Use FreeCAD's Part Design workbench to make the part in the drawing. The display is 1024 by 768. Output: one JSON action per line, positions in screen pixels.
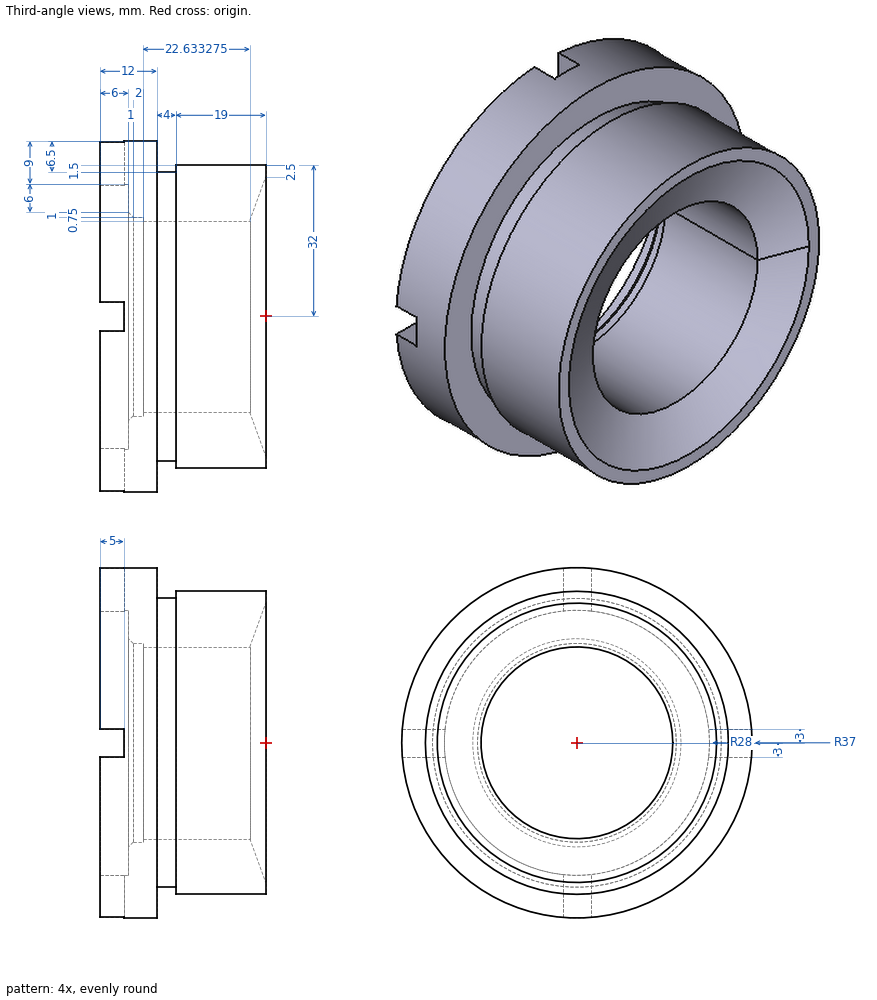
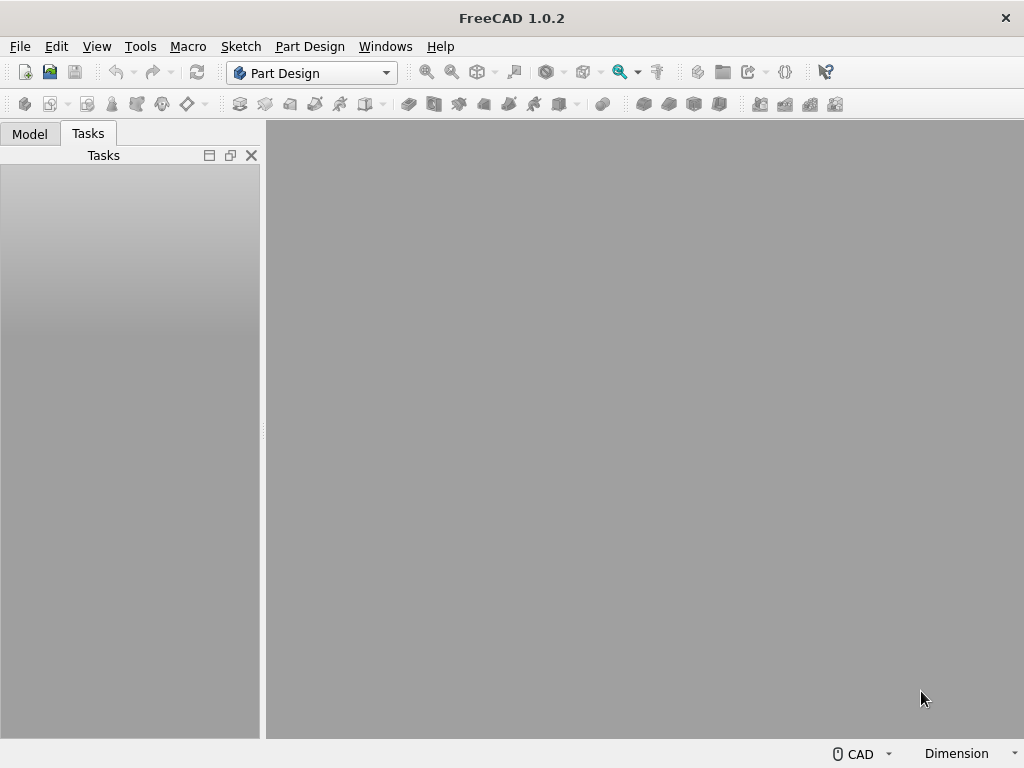
{"action": "left_click", "coordinate": [25, 72]}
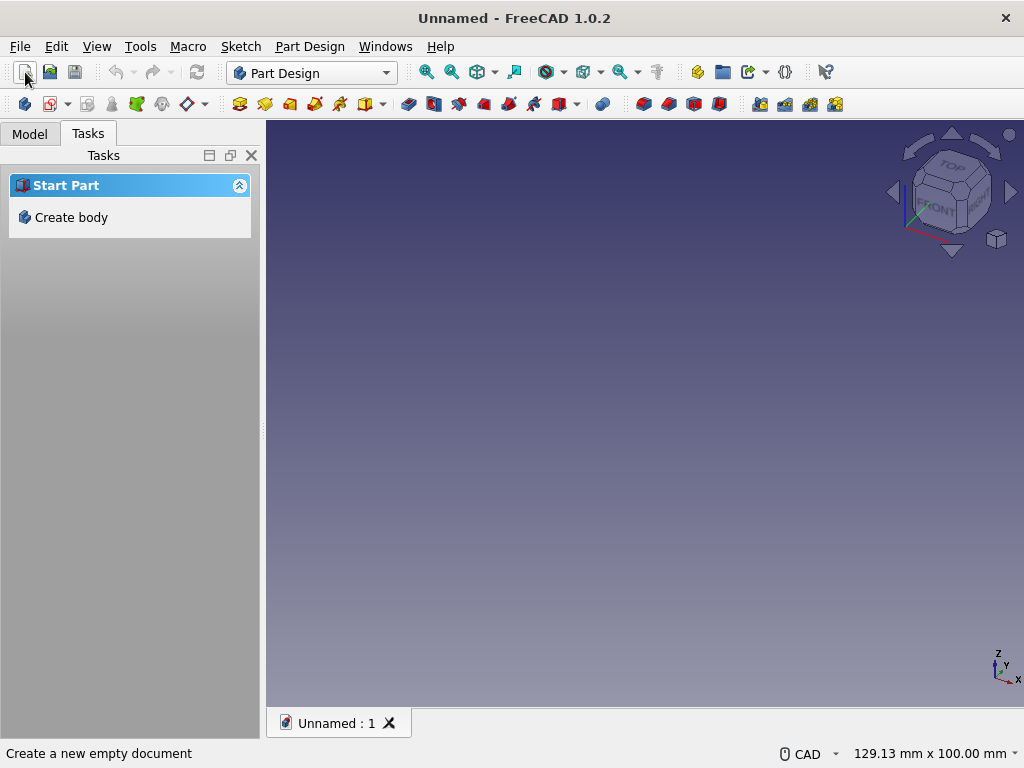
{"action": "left_click", "coordinate": [50, 104]}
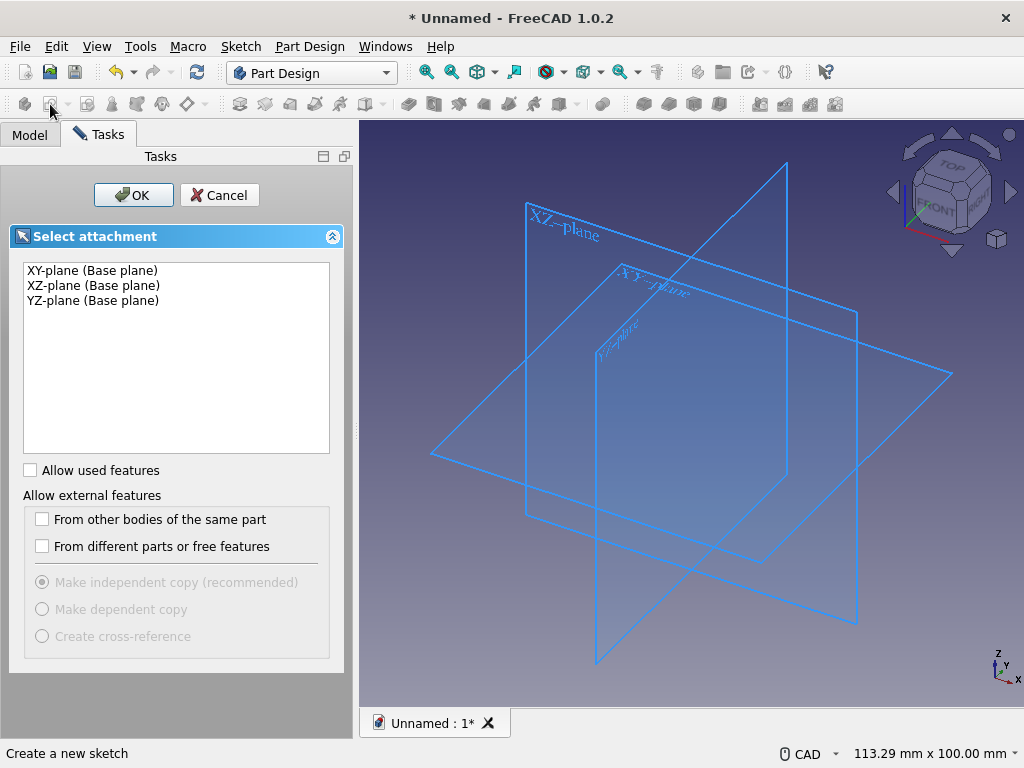
{"action": "left_click", "coordinate": [84, 270]}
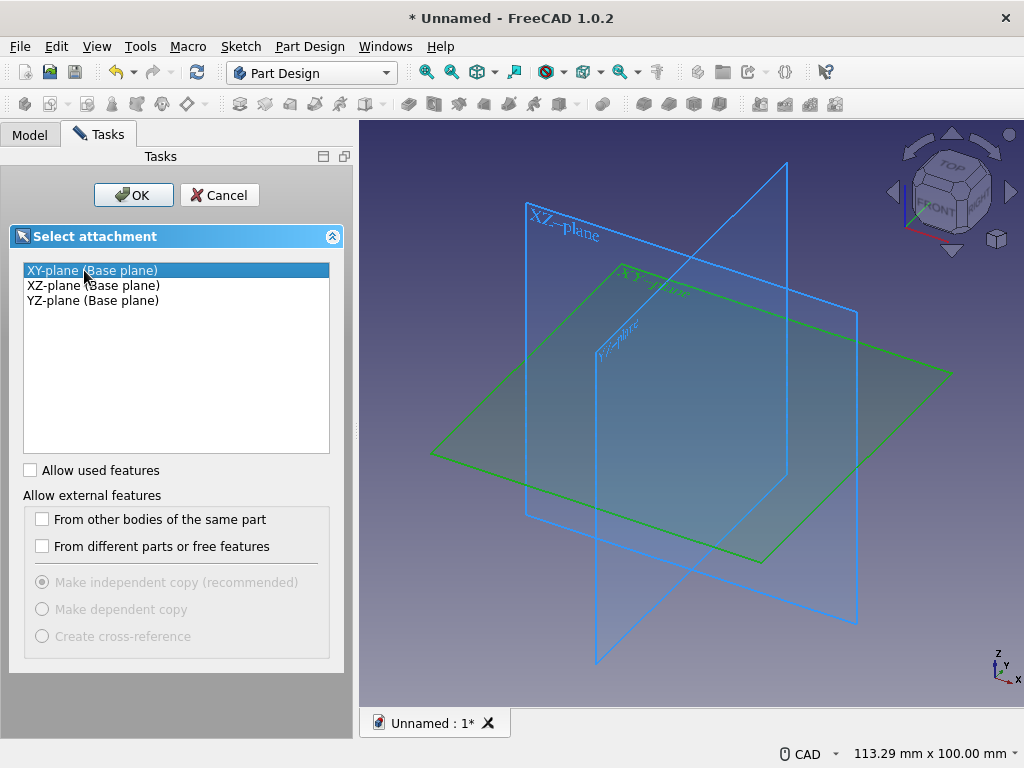
{"action": "left_click", "coordinate": [134, 195]}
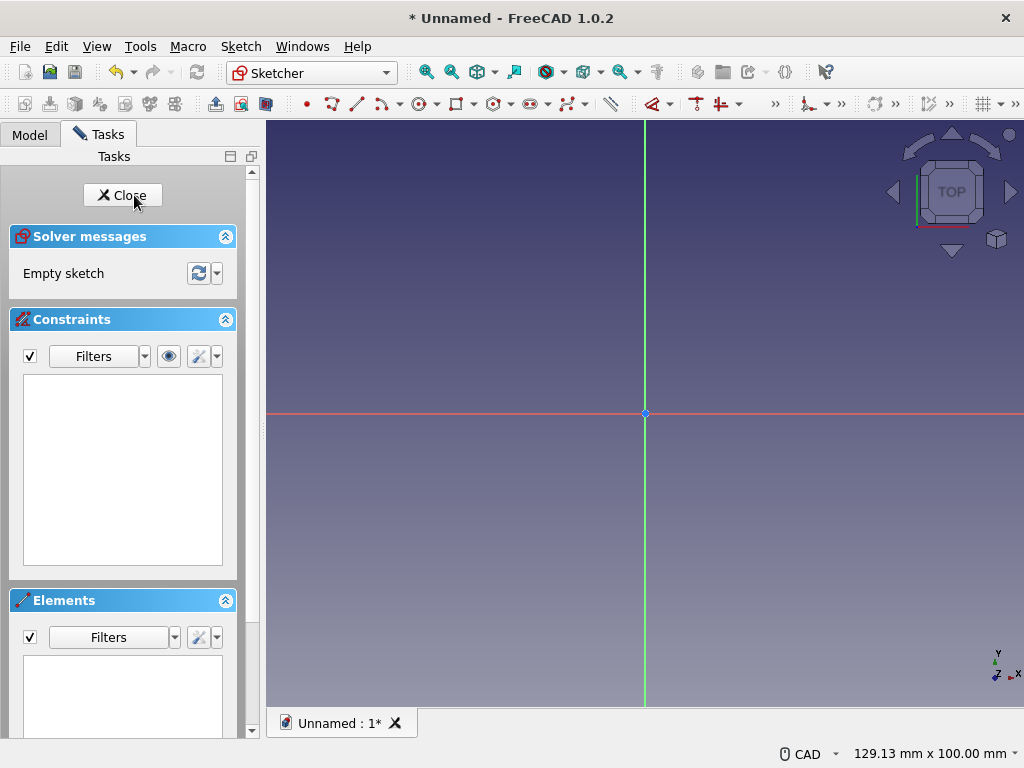
{"action": "scroll", "coordinate": [501, 173], "scroll_direction": "up", "scroll_amount": 3}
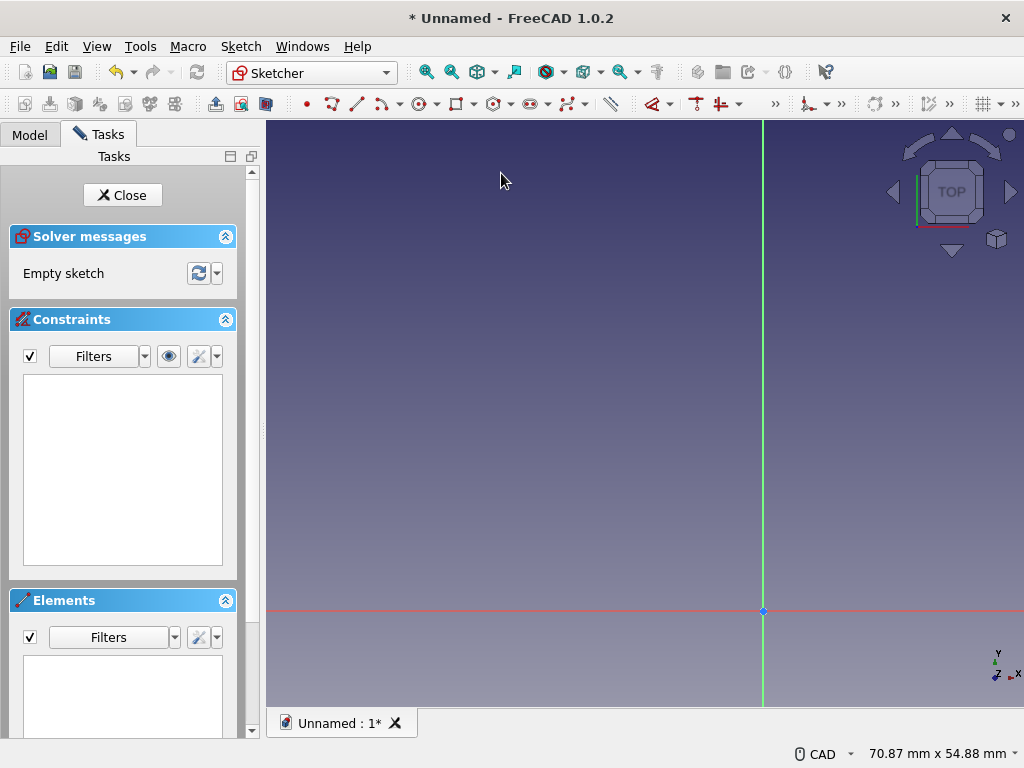
{"action": "left_click", "coordinate": [332, 104]}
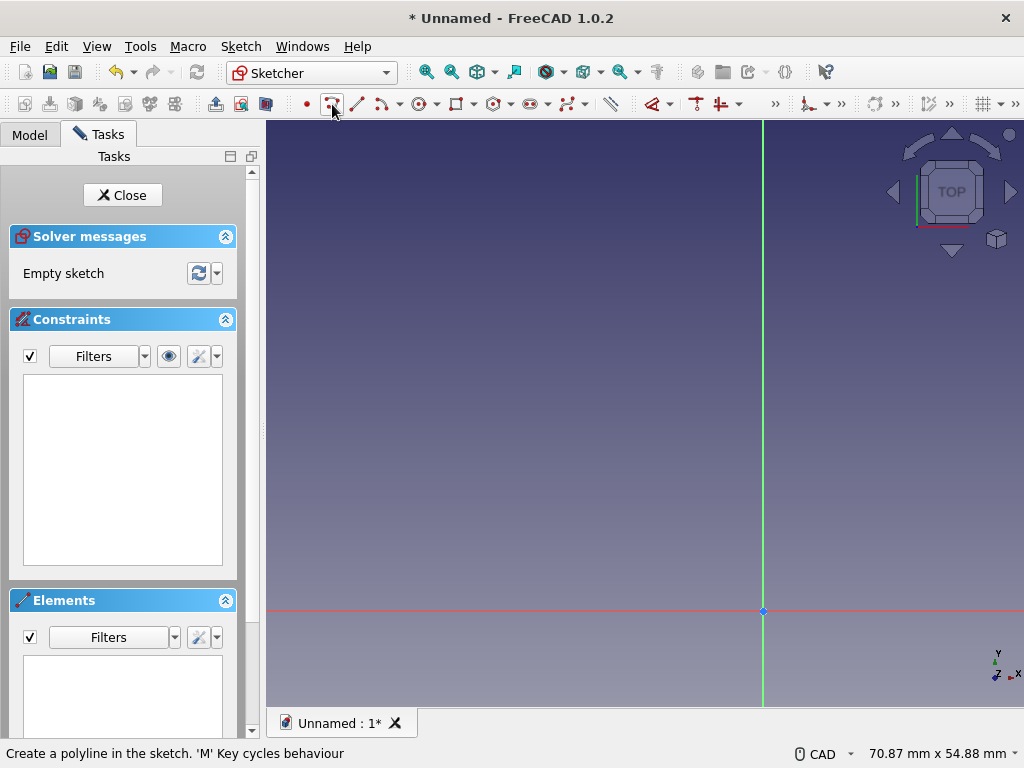
{"action": "left_click", "coordinate": [727, 395]}
{"action": "left_click", "coordinate": [763, 296]}
{"action": "left_click", "coordinate": [754, 269]}
{"action": "left_click", "coordinate": [560, 269]}
{"action": "left_click", "coordinate": [560, 285]}
{"action": "left_click", "coordinate": [517, 285]}
{"action": "left_click", "coordinate": [517, 215]}
{"action": "left_click", "coordinate": [389, 215]}
{"action": "left_click", "coordinate": [389, 312]}
{"action": "left_click", "coordinate": [453, 312]}
{"action": "left_click", "coordinate": [453, 376]}
{"action": "left_click", "coordinate": [464, 387]}
{"action": "left_click", "coordinate": [485, 387]}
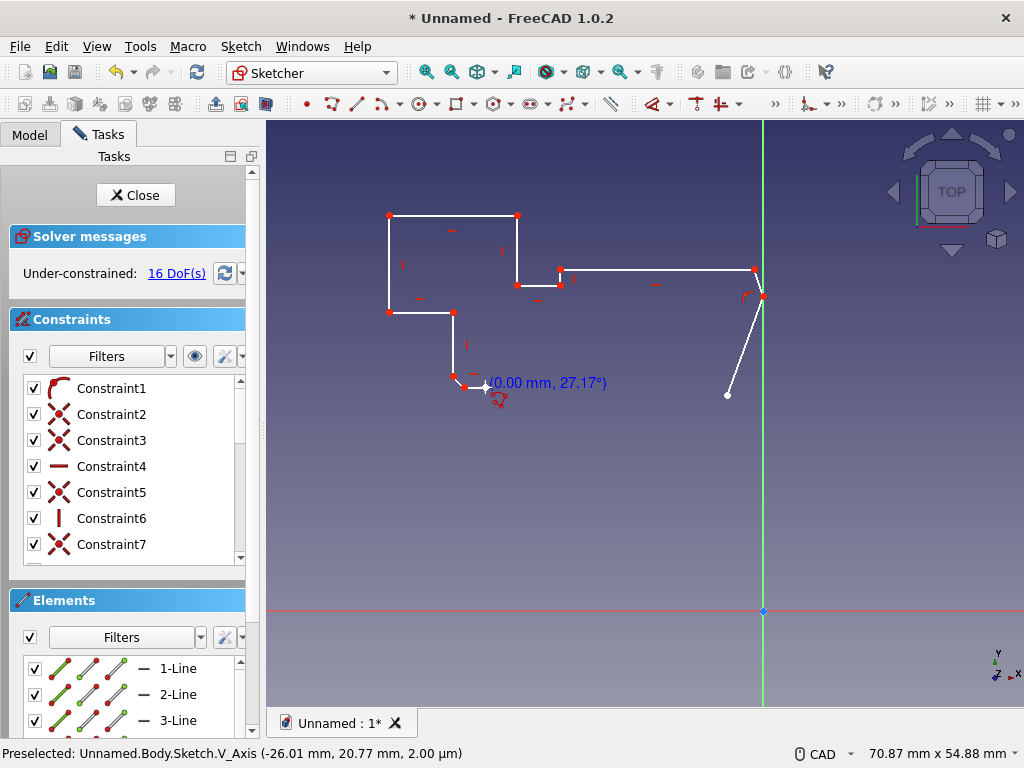
{"action": "scroll", "coordinate": [485, 395], "scroll_direction": "up", "scroll_amount": 4}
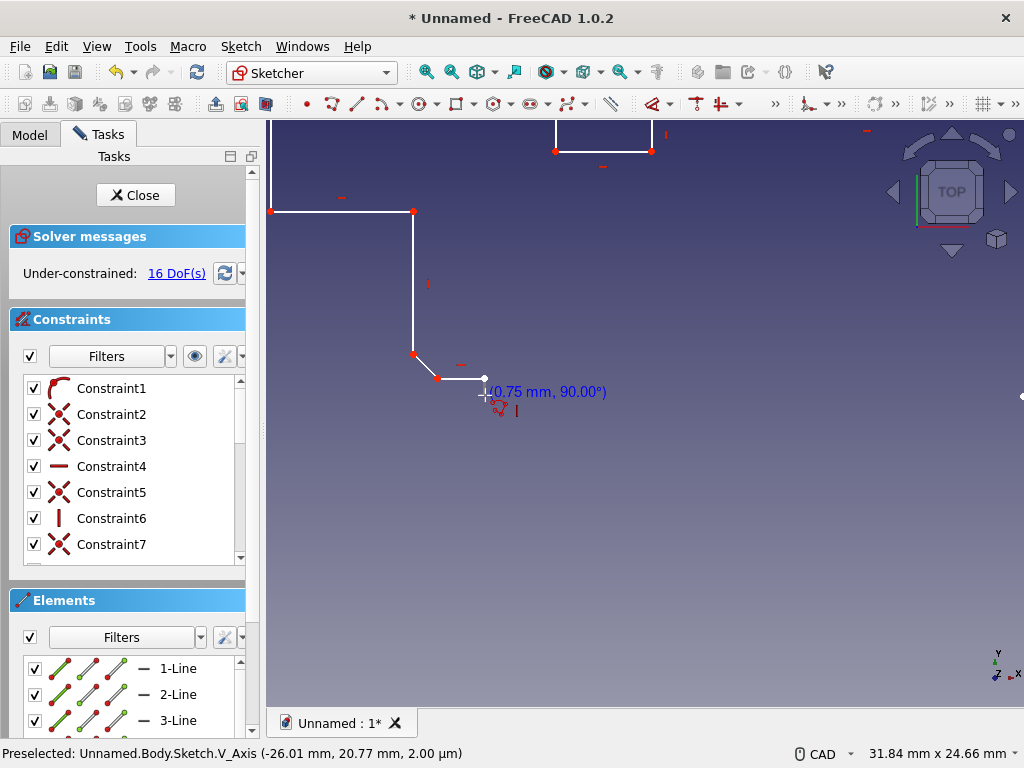
{"action": "left_click", "coordinate": [485, 393]}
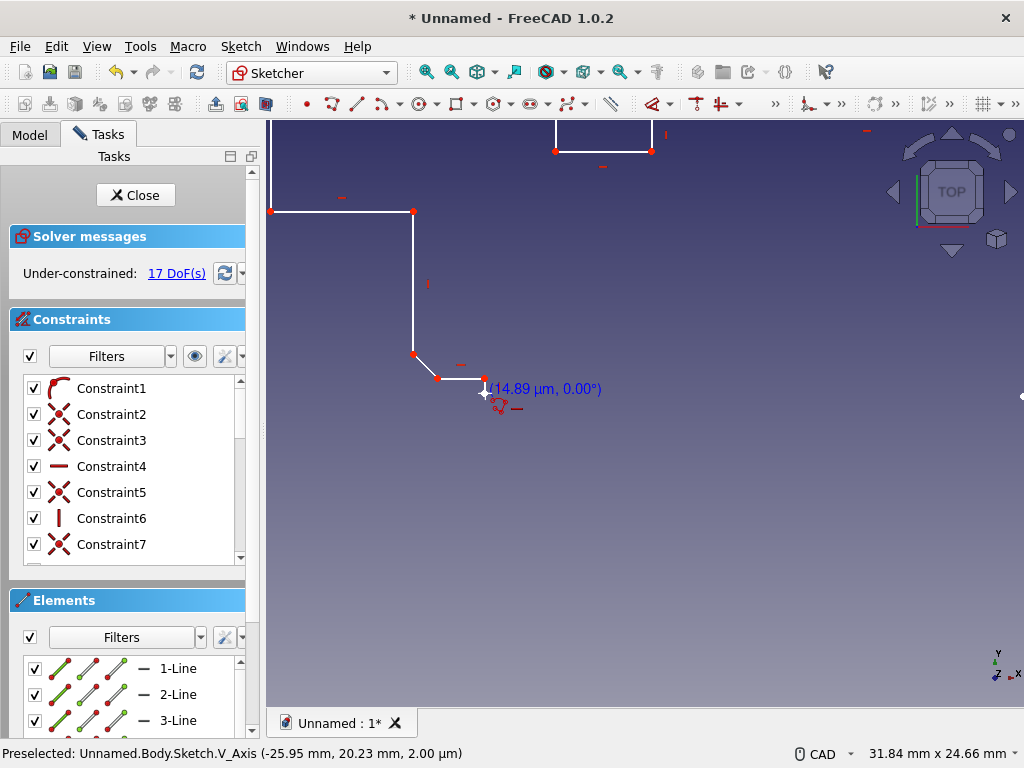
{"action": "scroll", "coordinate": [486, 396], "scroll_direction": "down", "scroll_amount": 4}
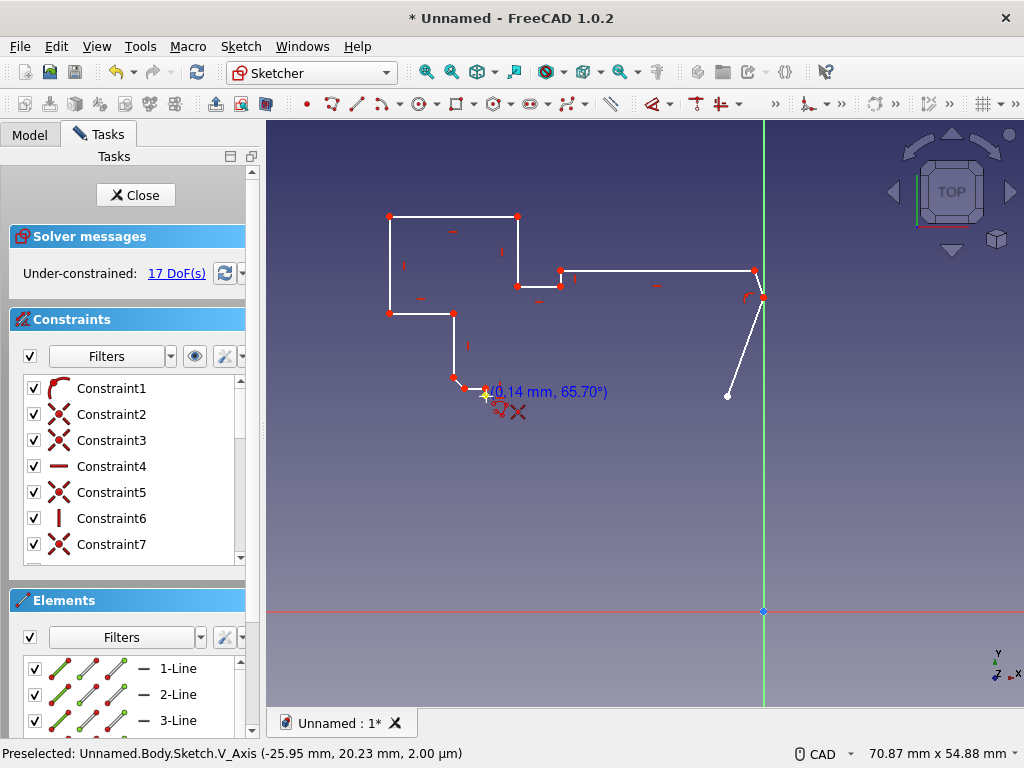
{"action": "left_click", "coordinate": [728, 397]}
{"action": "key", "text": "Escape"}
{"action": "key", "text": "Escape"}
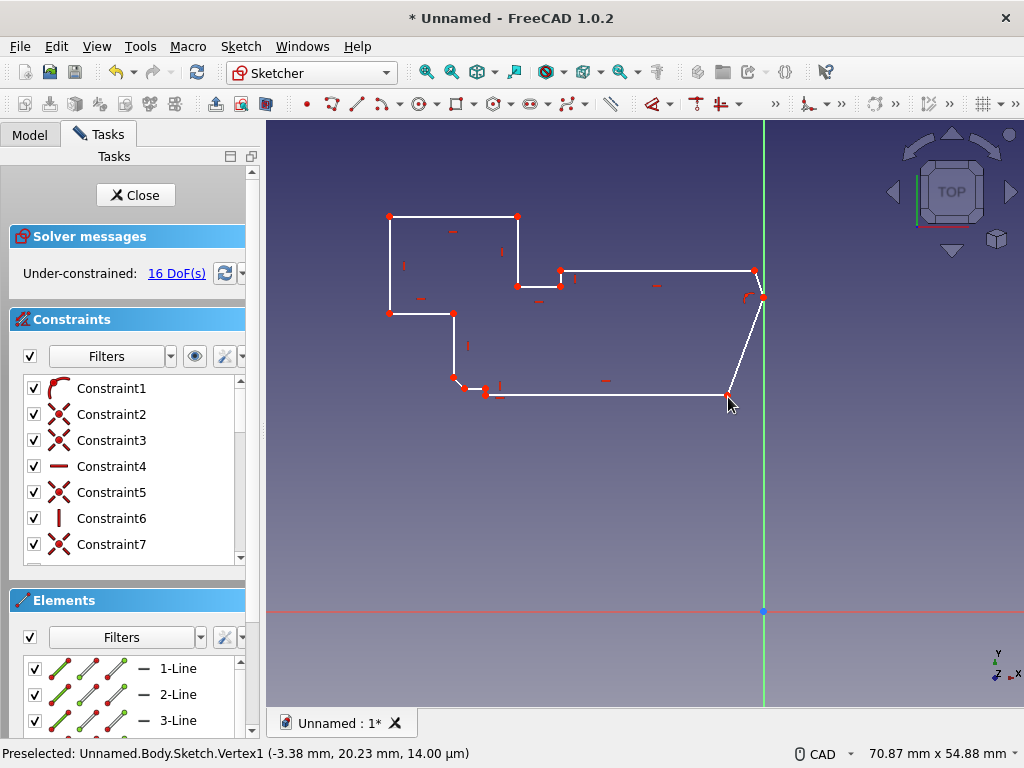
{"action": "left_click", "coordinate": [760, 287]}